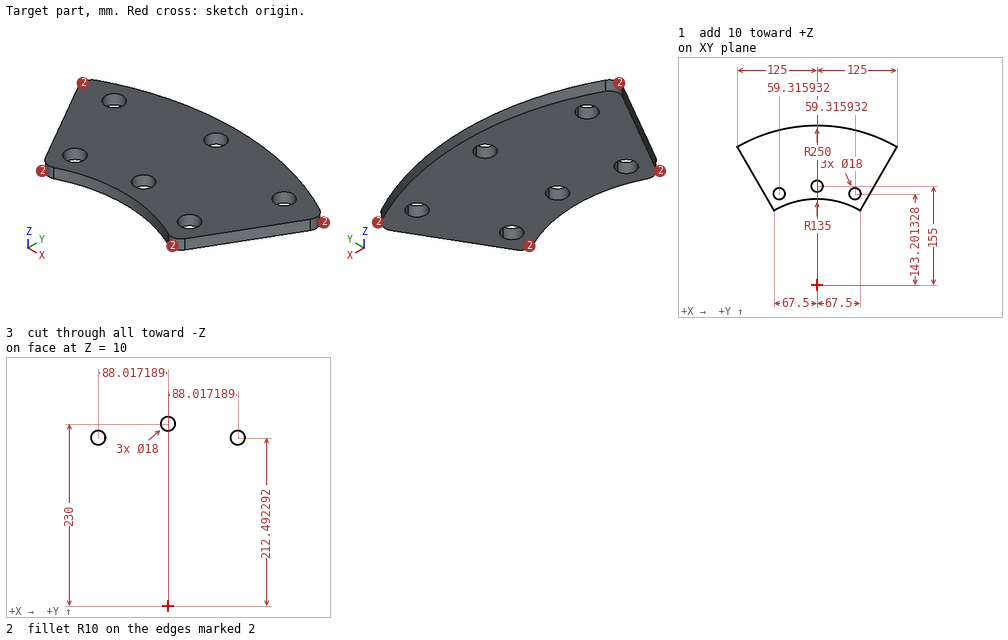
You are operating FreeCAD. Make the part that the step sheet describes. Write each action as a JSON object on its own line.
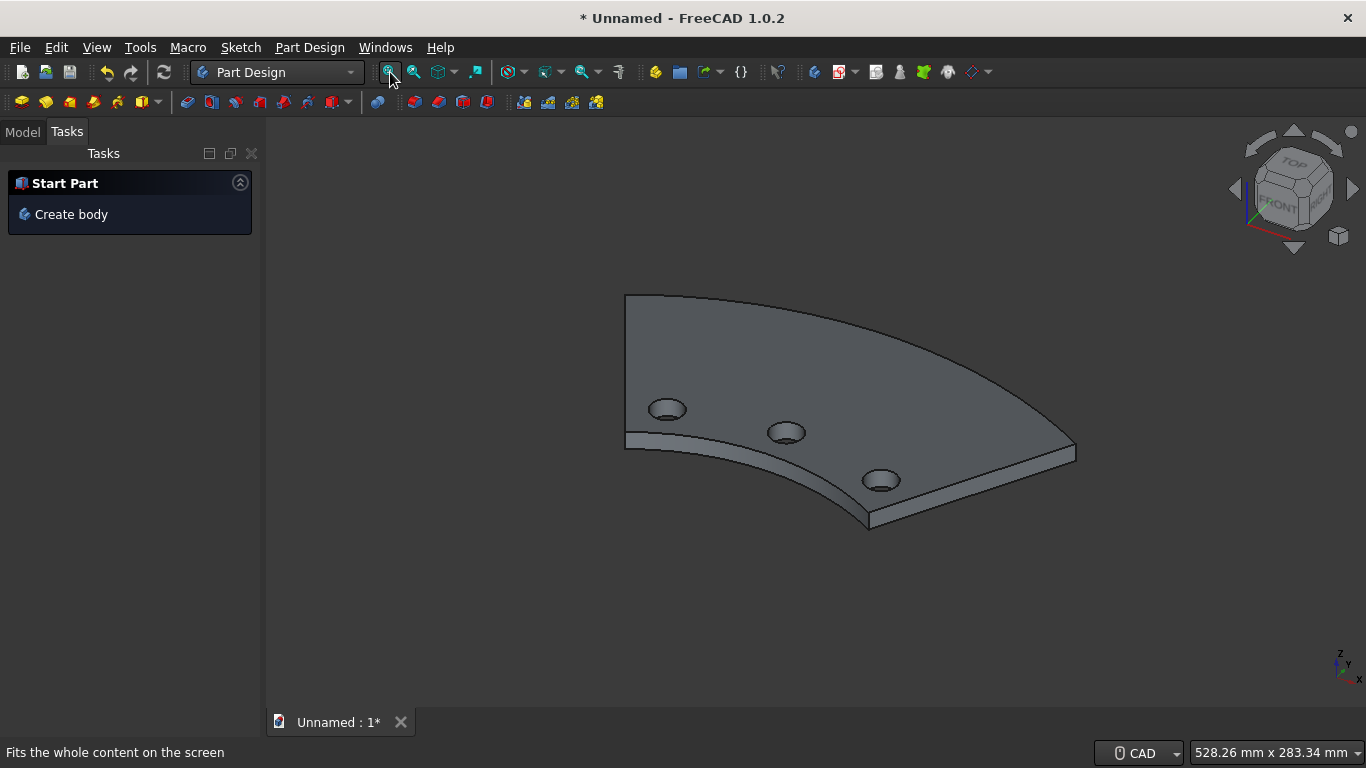
{"action": "left_click", "coordinate": [869, 520]}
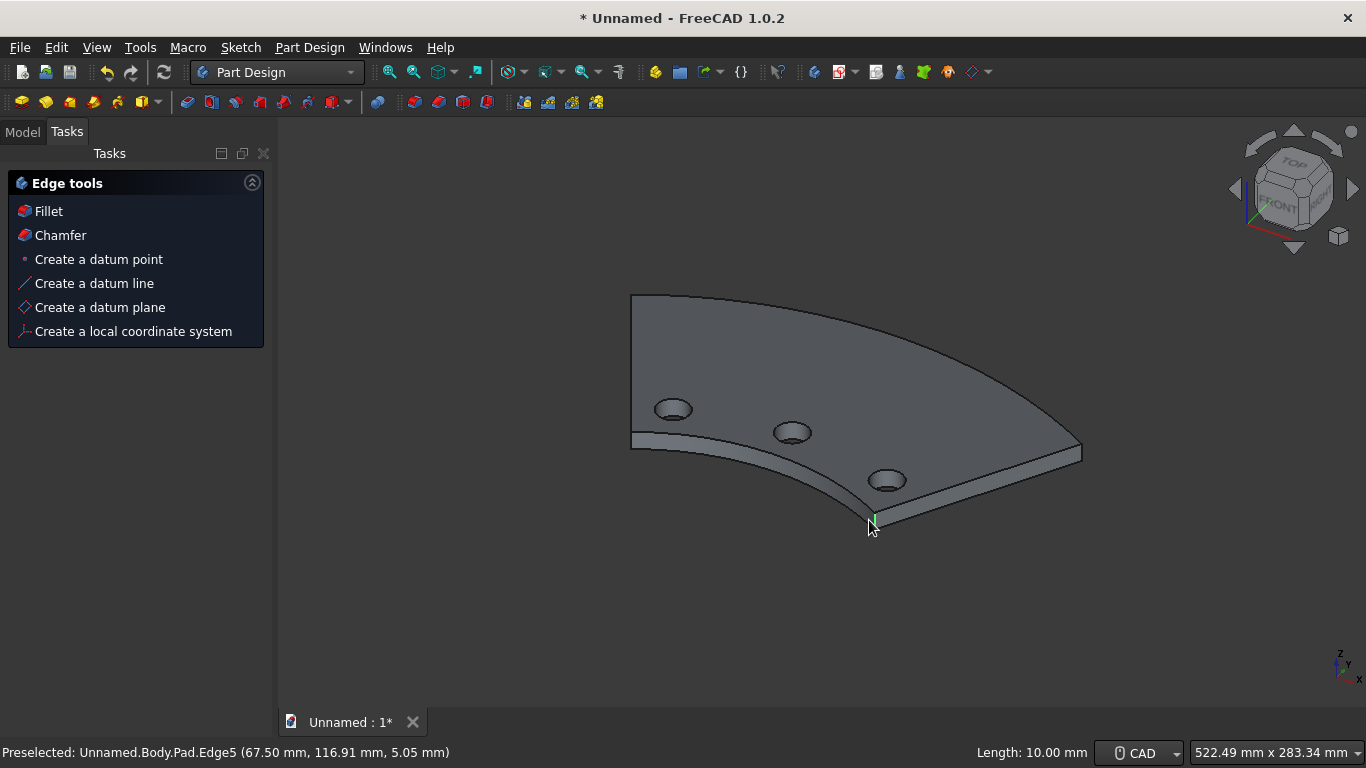
{"action": "scroll", "coordinate": [631, 439], "scroll_direction": "up", "scroll_amount": 4}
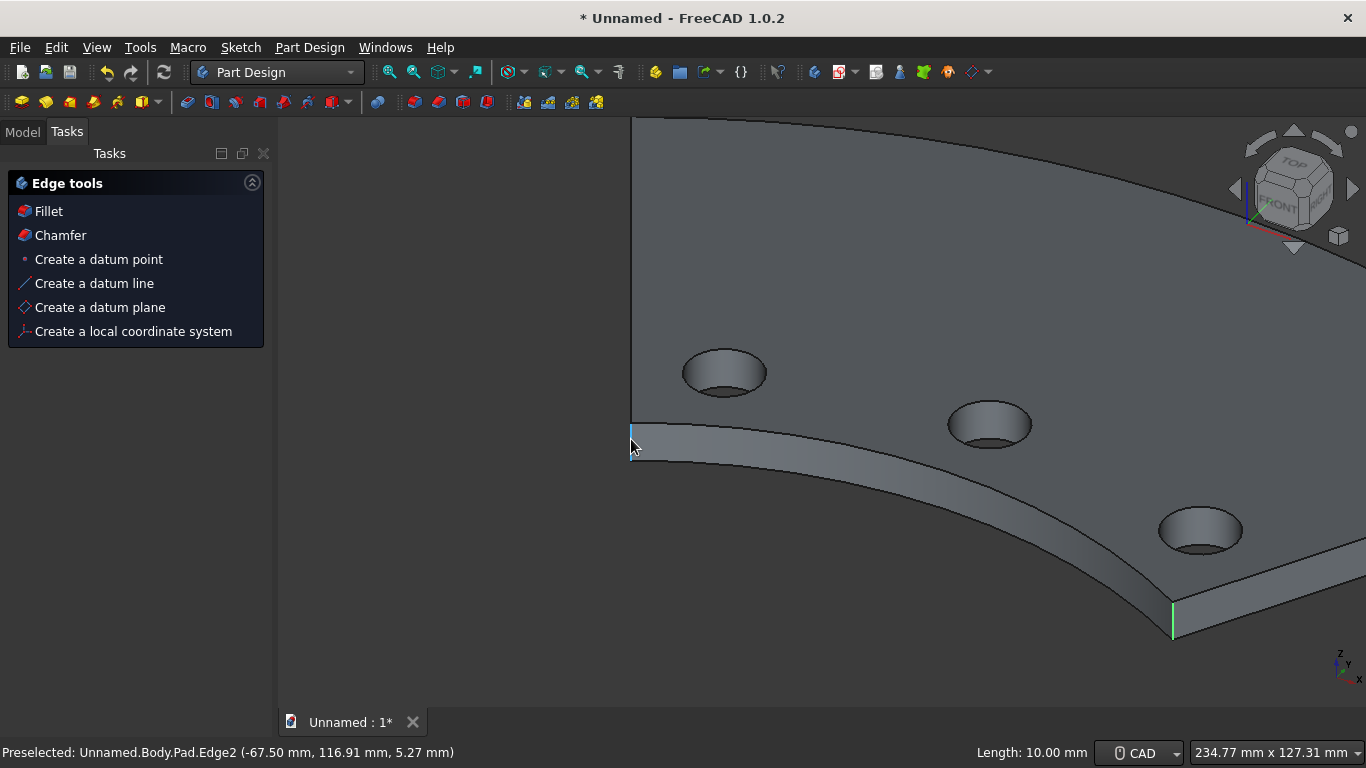
{"action": "left_click", "coordinate": [390, 72]}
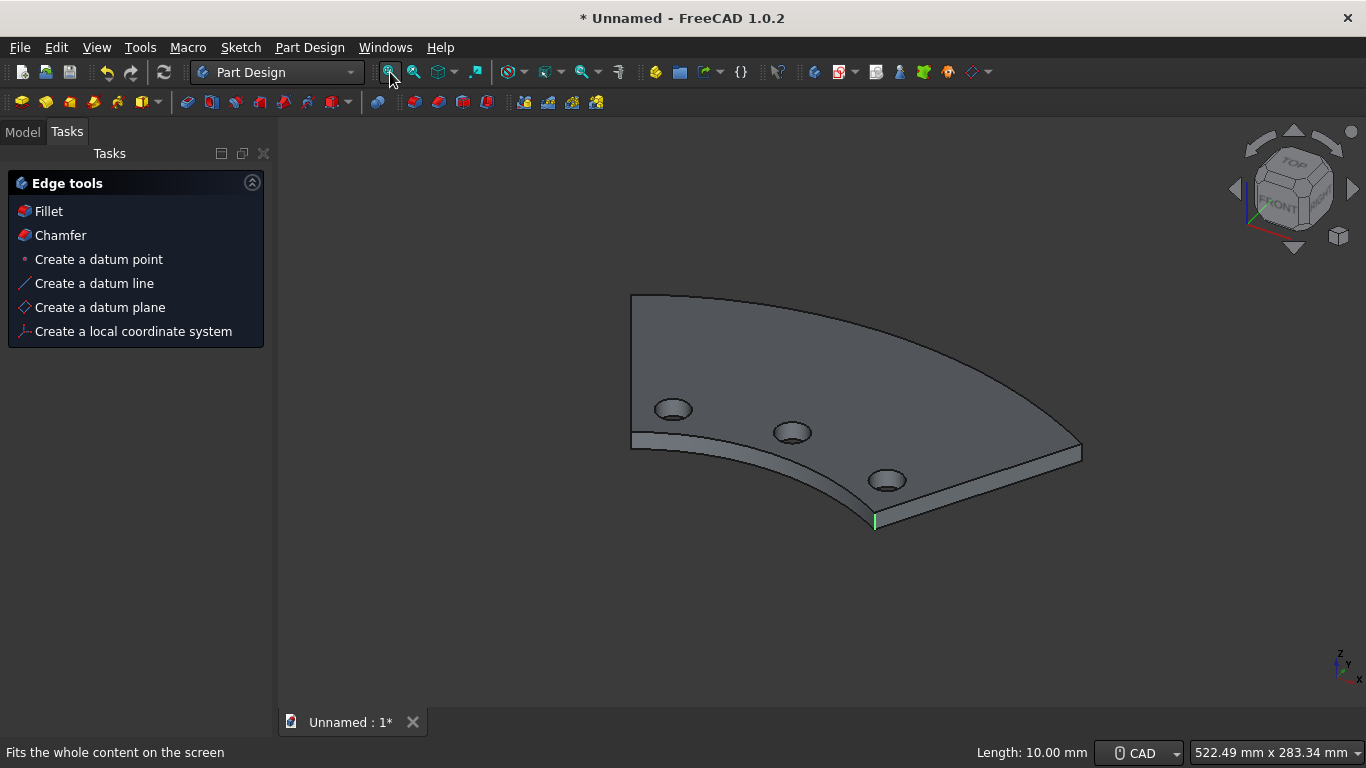
{"action": "key", "text": "0"}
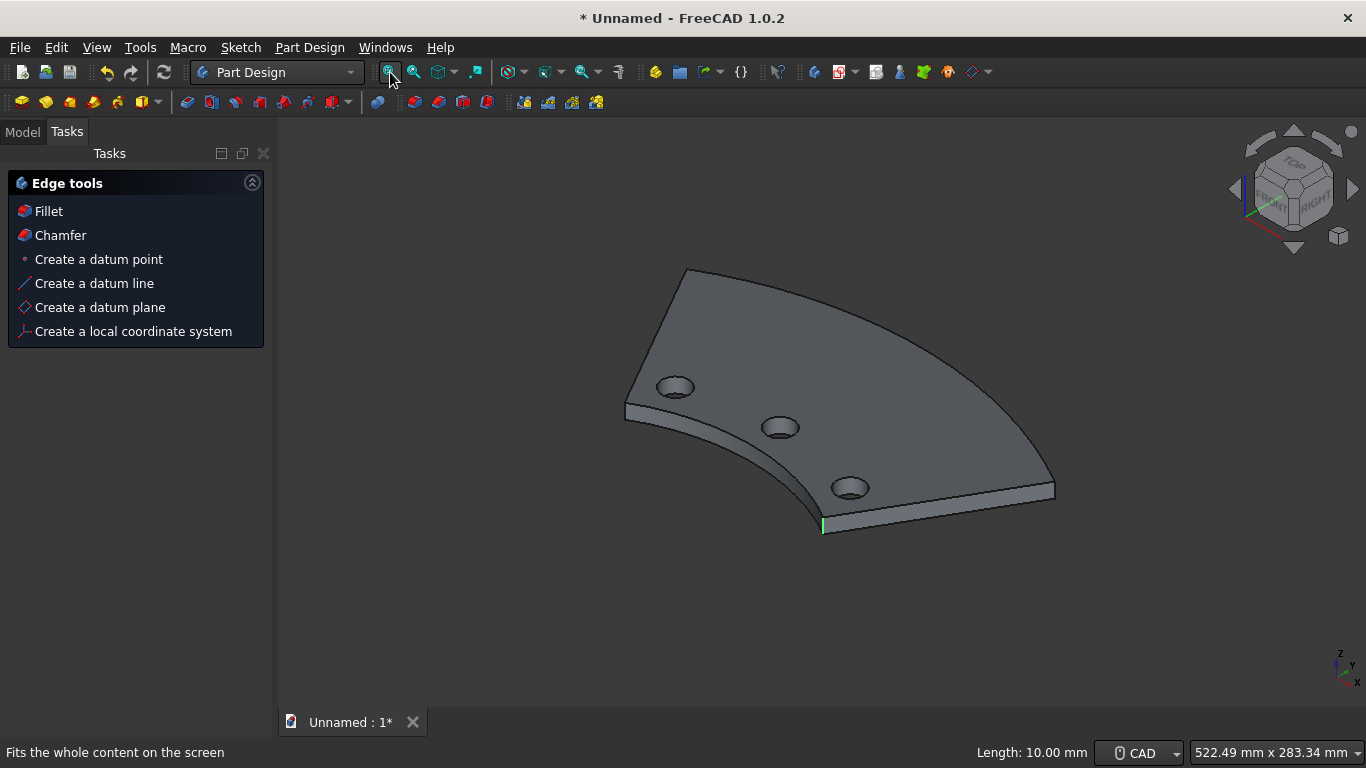
{"action": "scroll", "coordinate": [625, 410], "scroll_direction": "up", "scroll_amount": 4}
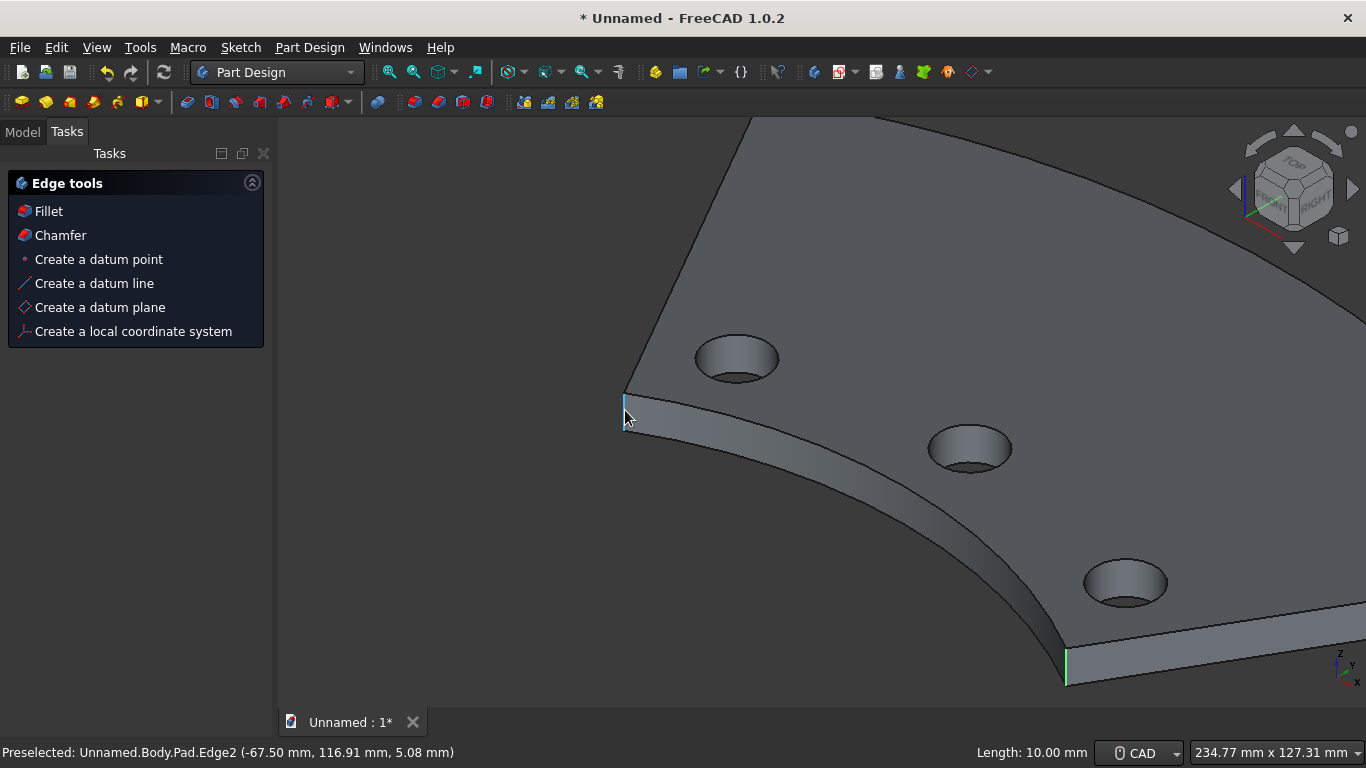
{"action": "left_click", "coordinate": [390, 72]}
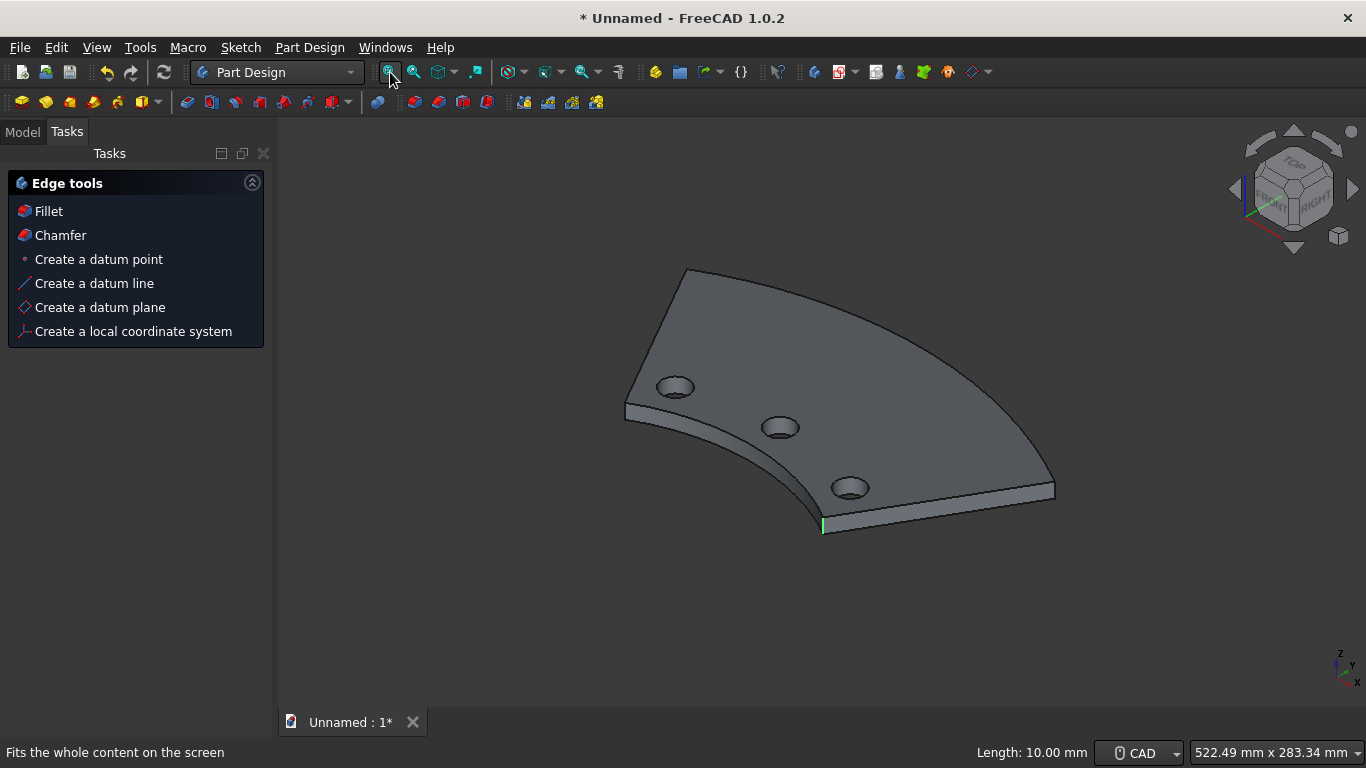
{"action": "key", "text": "2"}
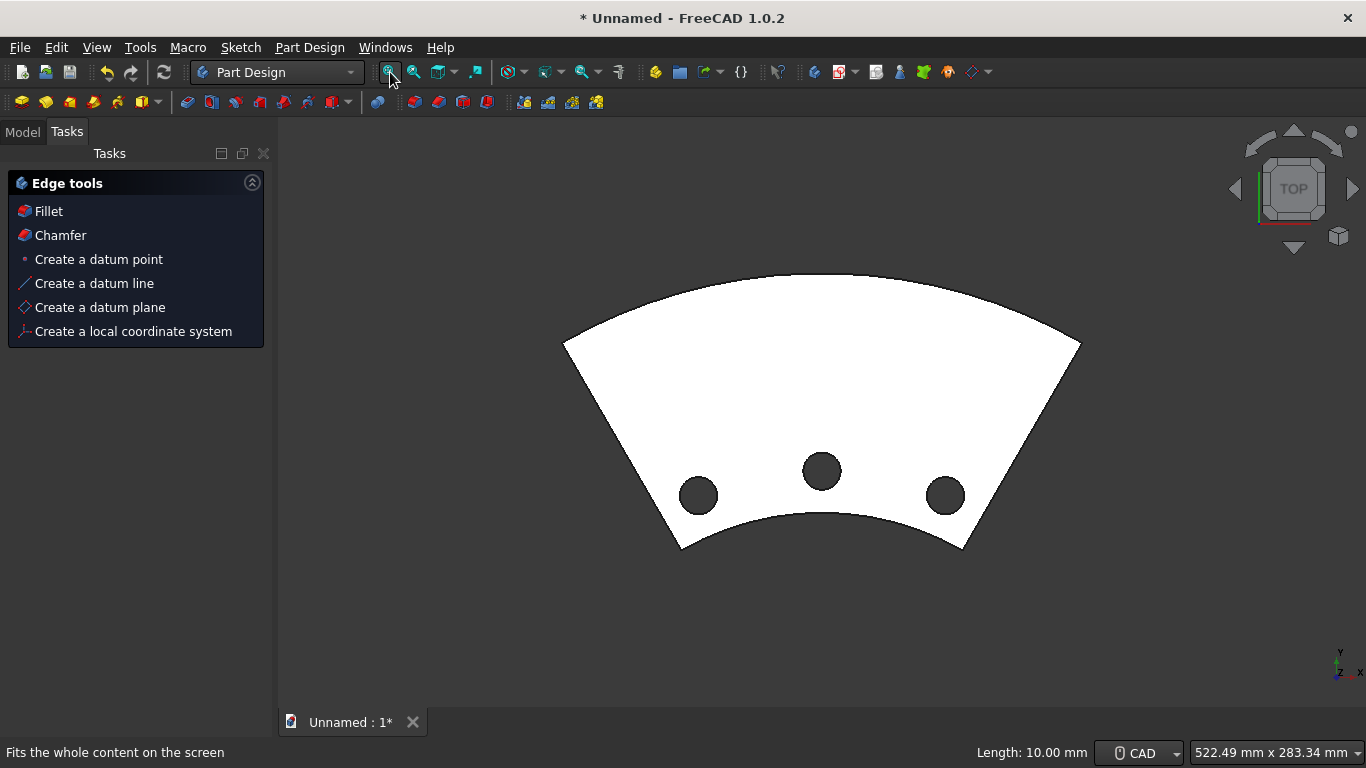
{"action": "scroll", "coordinate": [681, 549], "scroll_direction": "up", "scroll_amount": 4}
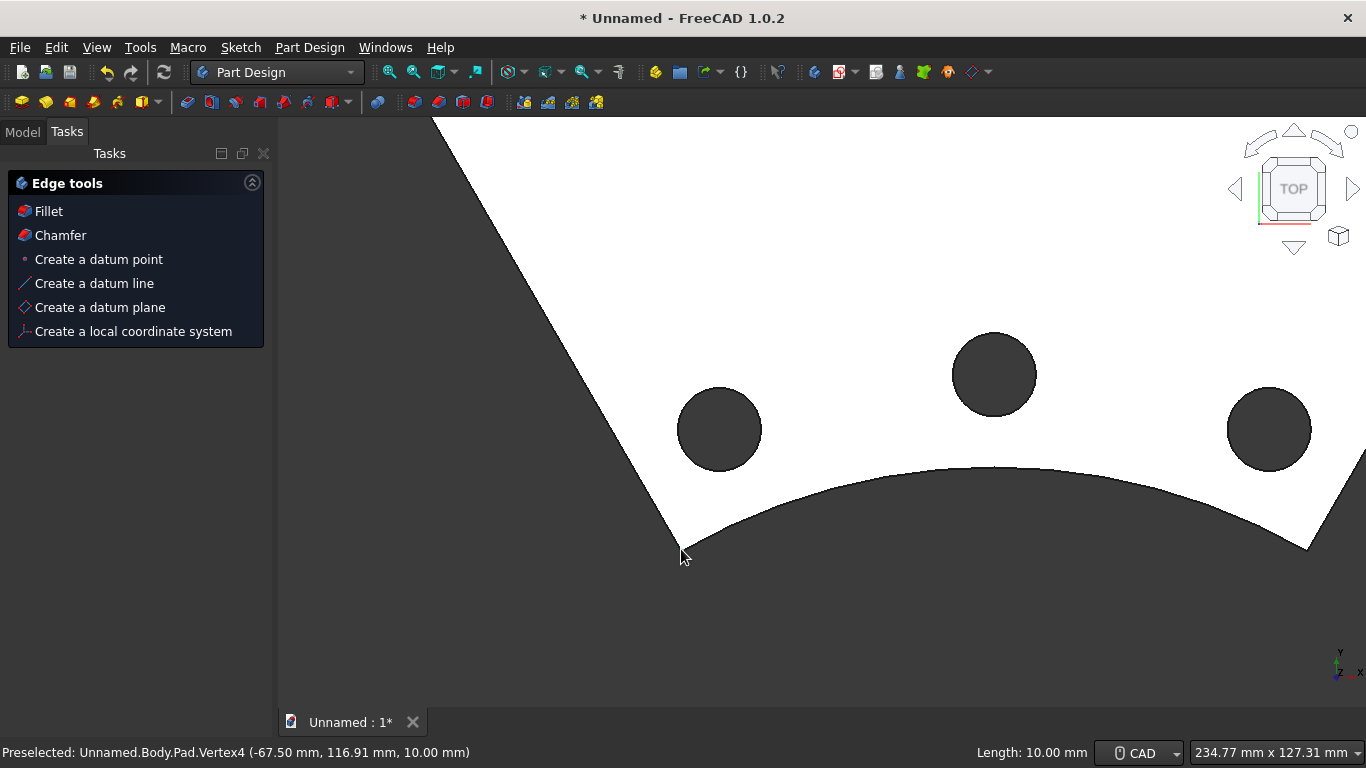
{"action": "left_click", "coordinate": [390, 72]}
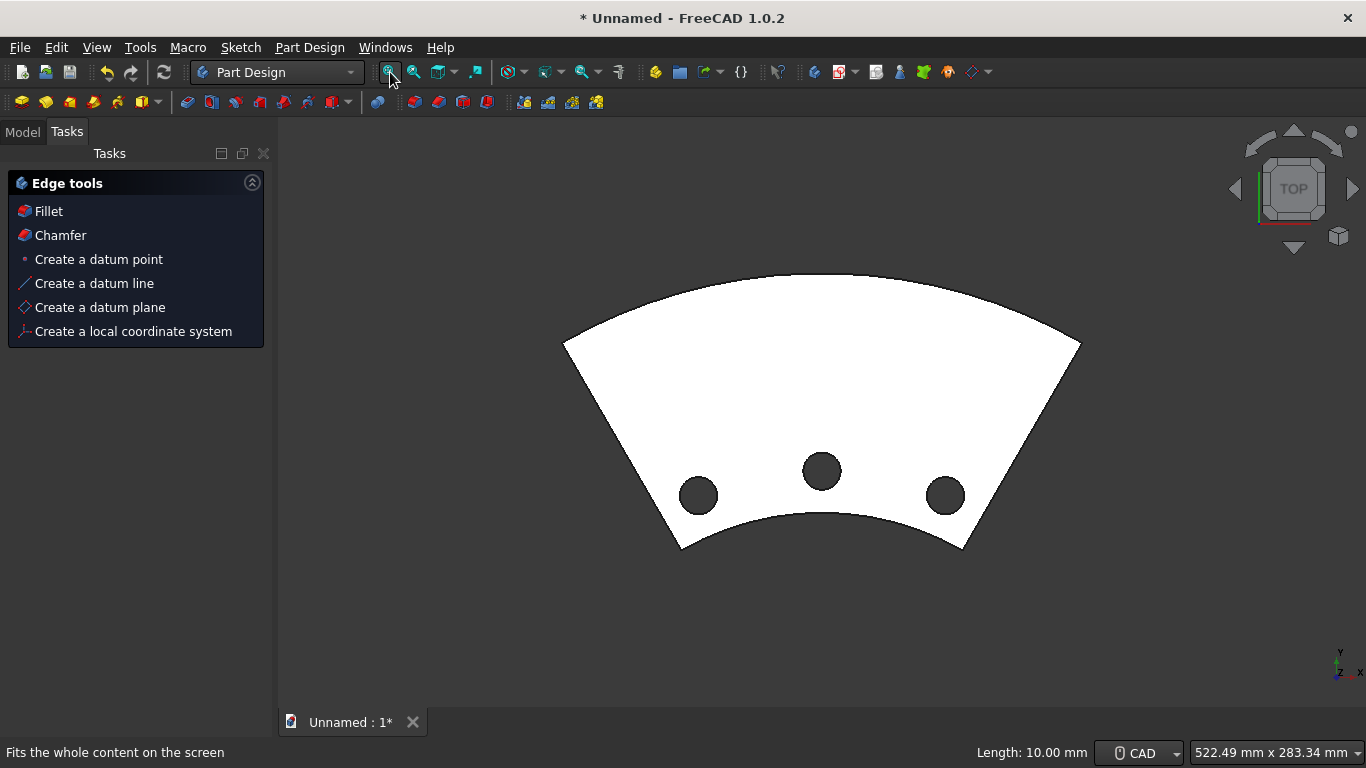
{"action": "key", "text": "1"}